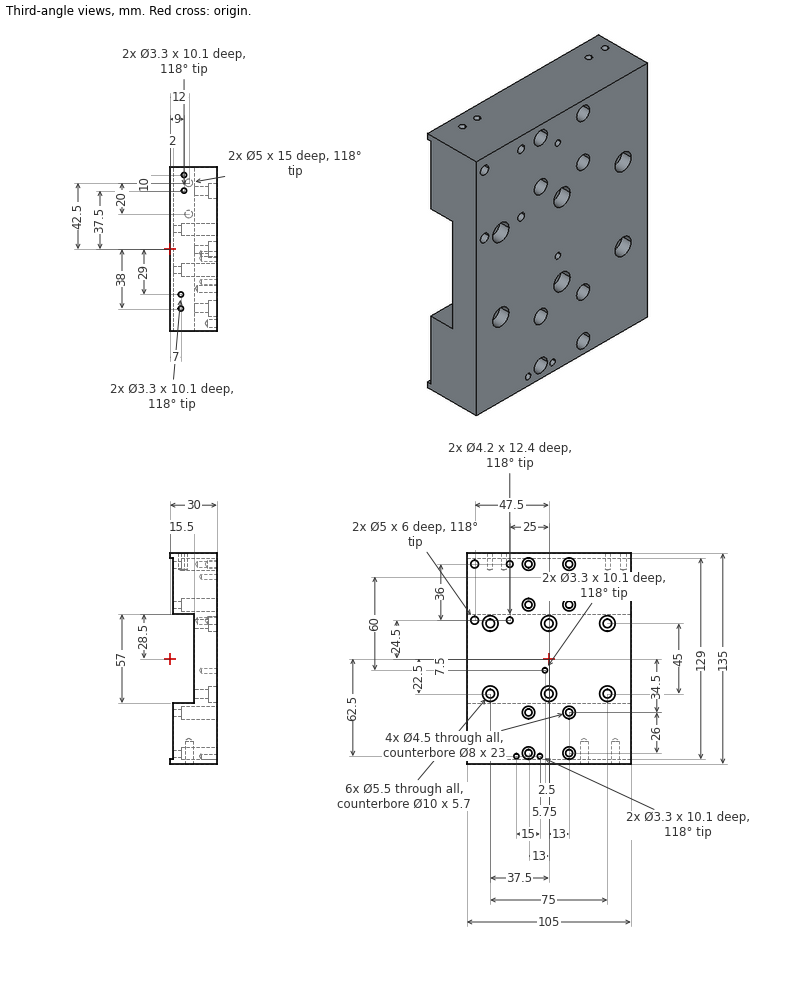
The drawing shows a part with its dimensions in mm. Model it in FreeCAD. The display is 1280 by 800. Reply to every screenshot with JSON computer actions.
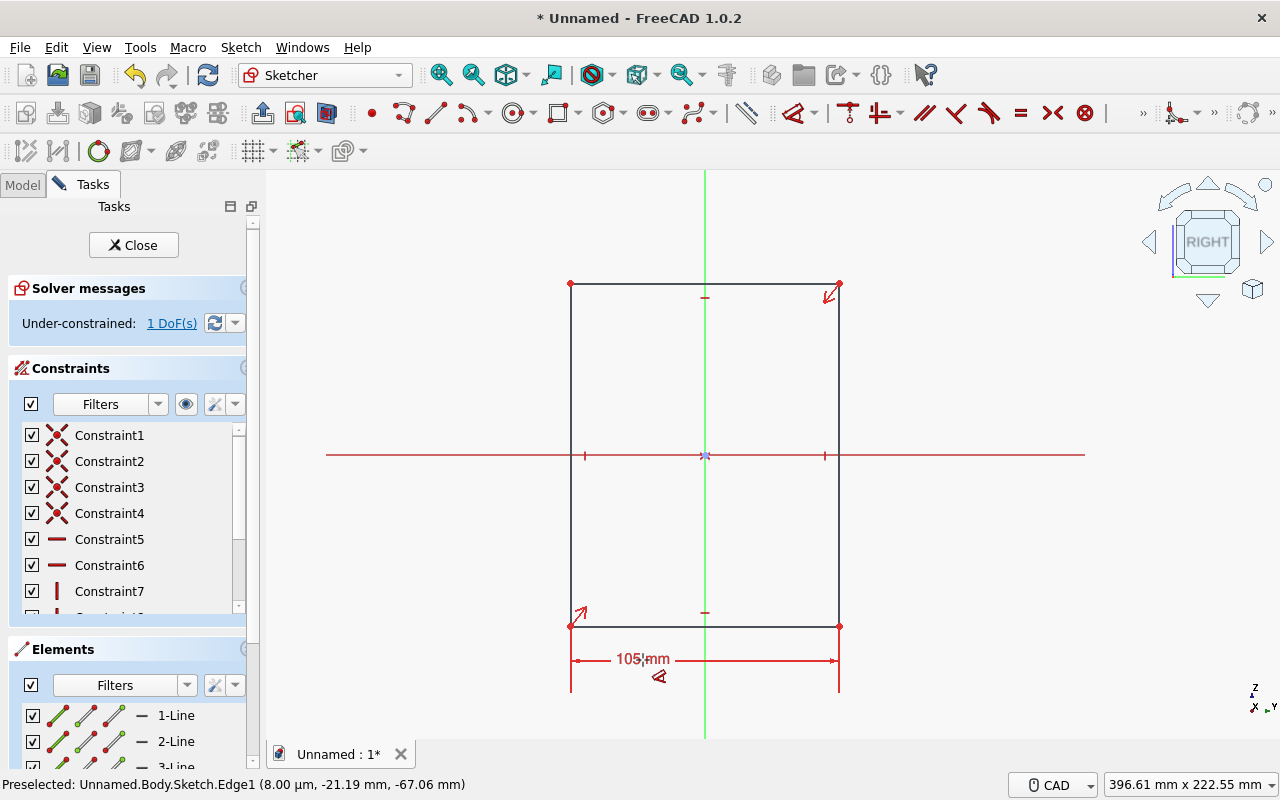
{"action": "left_click", "coordinate": [839, 524]}
{"action": "left_click", "coordinate": [873, 376]}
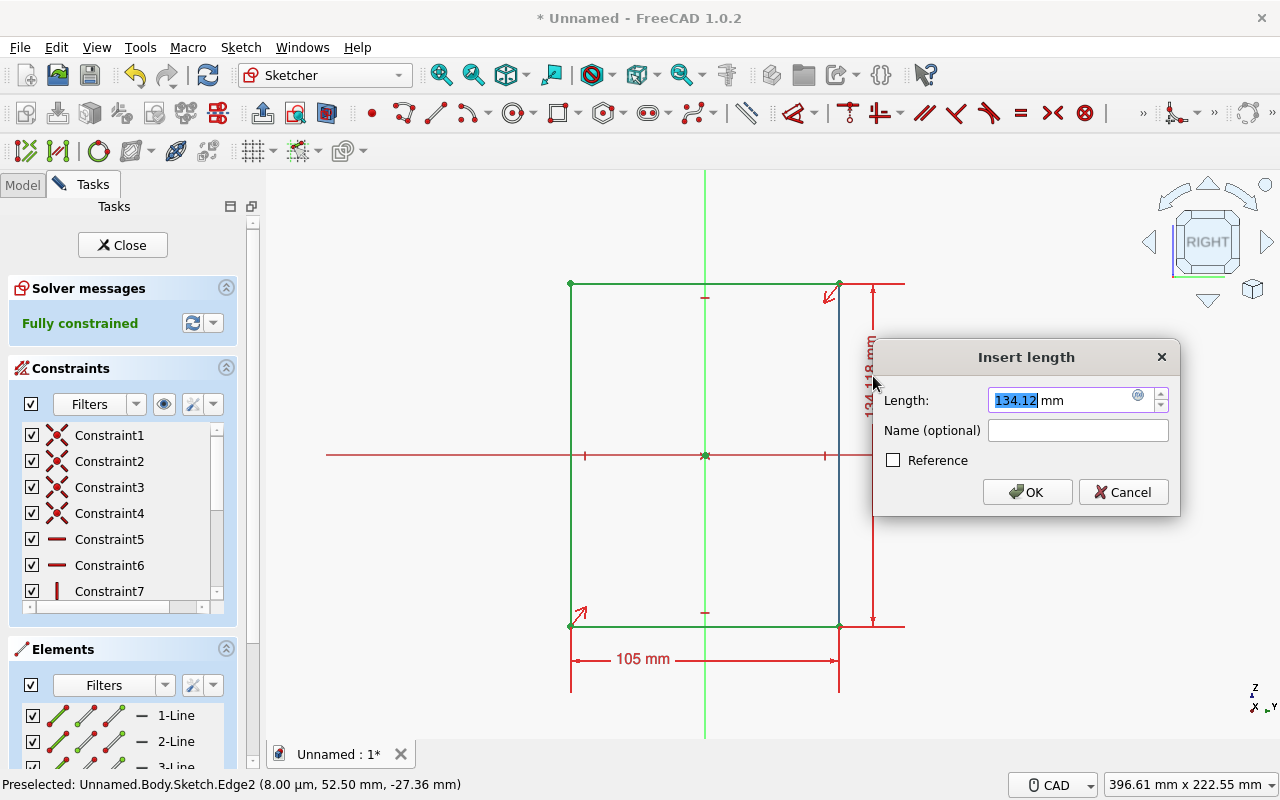
{"action": "type", "text": "135"}
{"action": "key", "text": "Return"}
{"action": "key", "text": "Escape"}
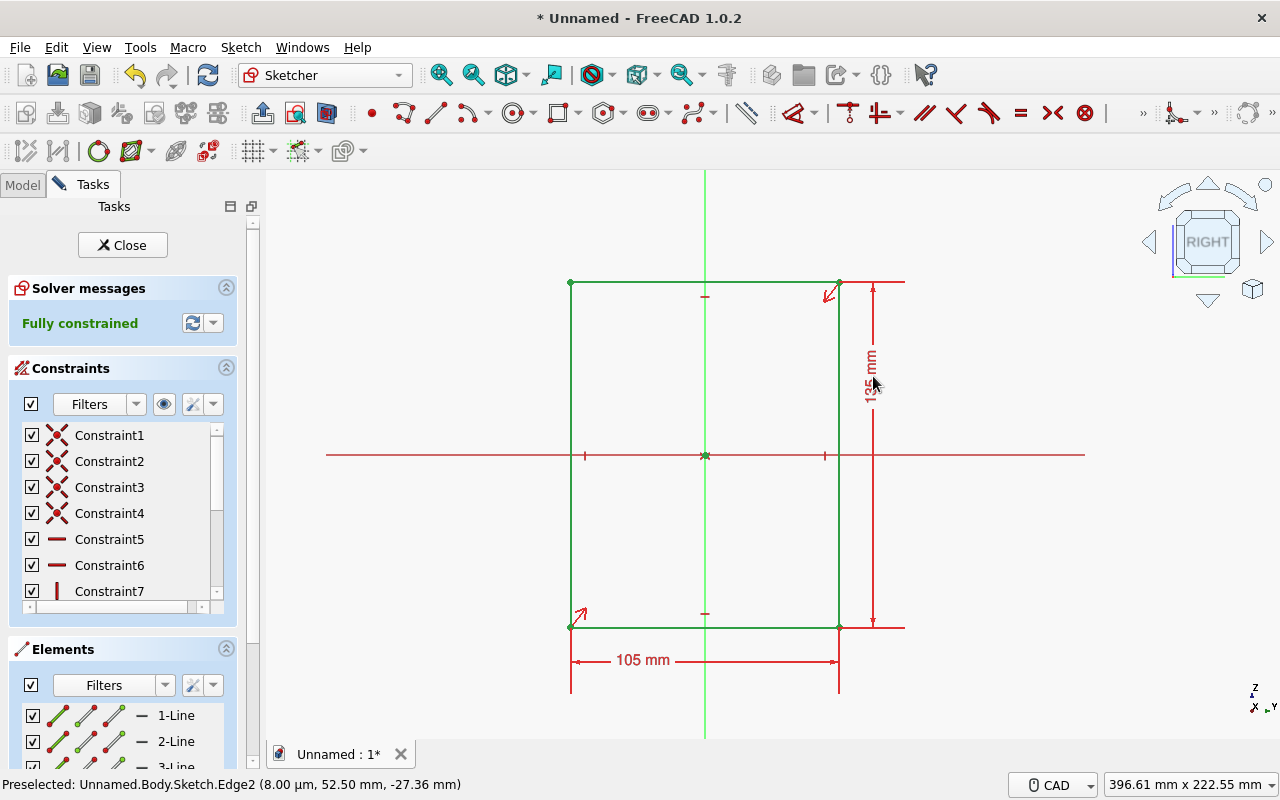
{"action": "left_click", "coordinate": [123, 245]}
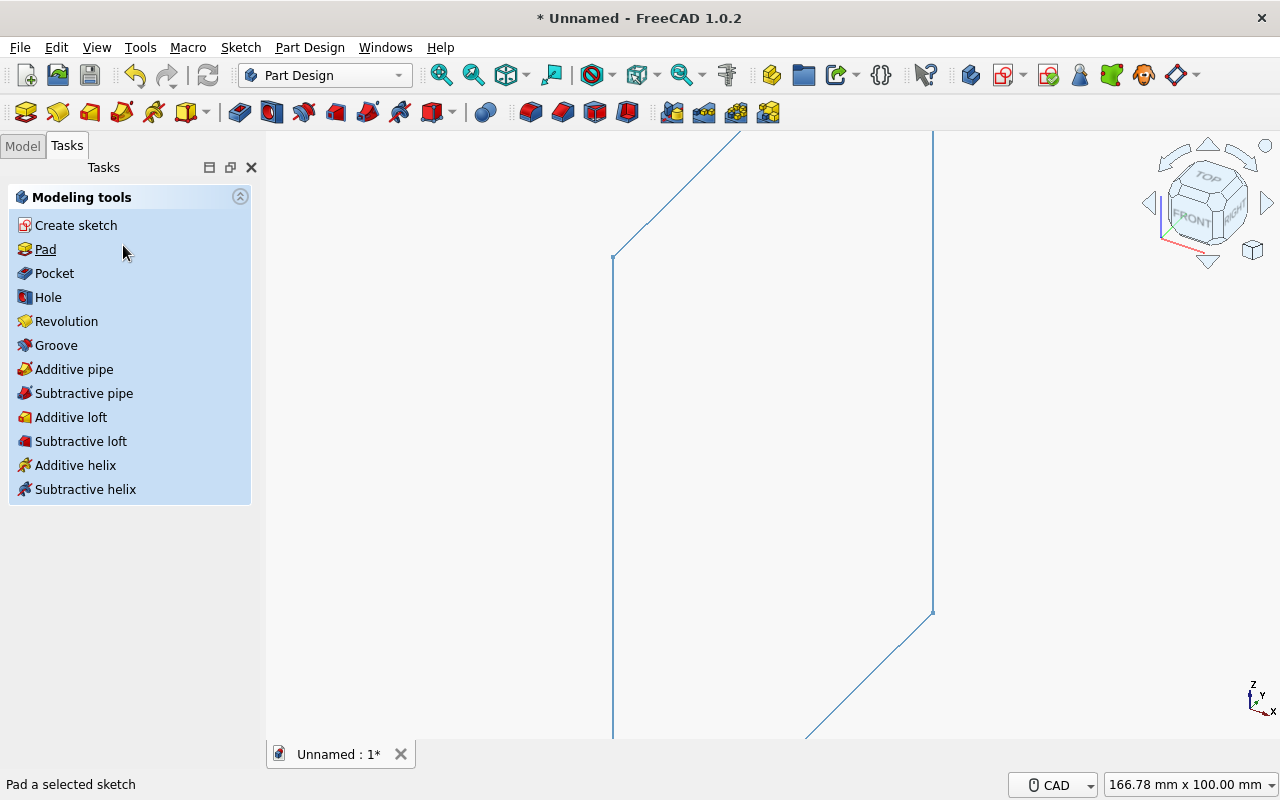
{"action": "left_click", "coordinate": [26, 112]}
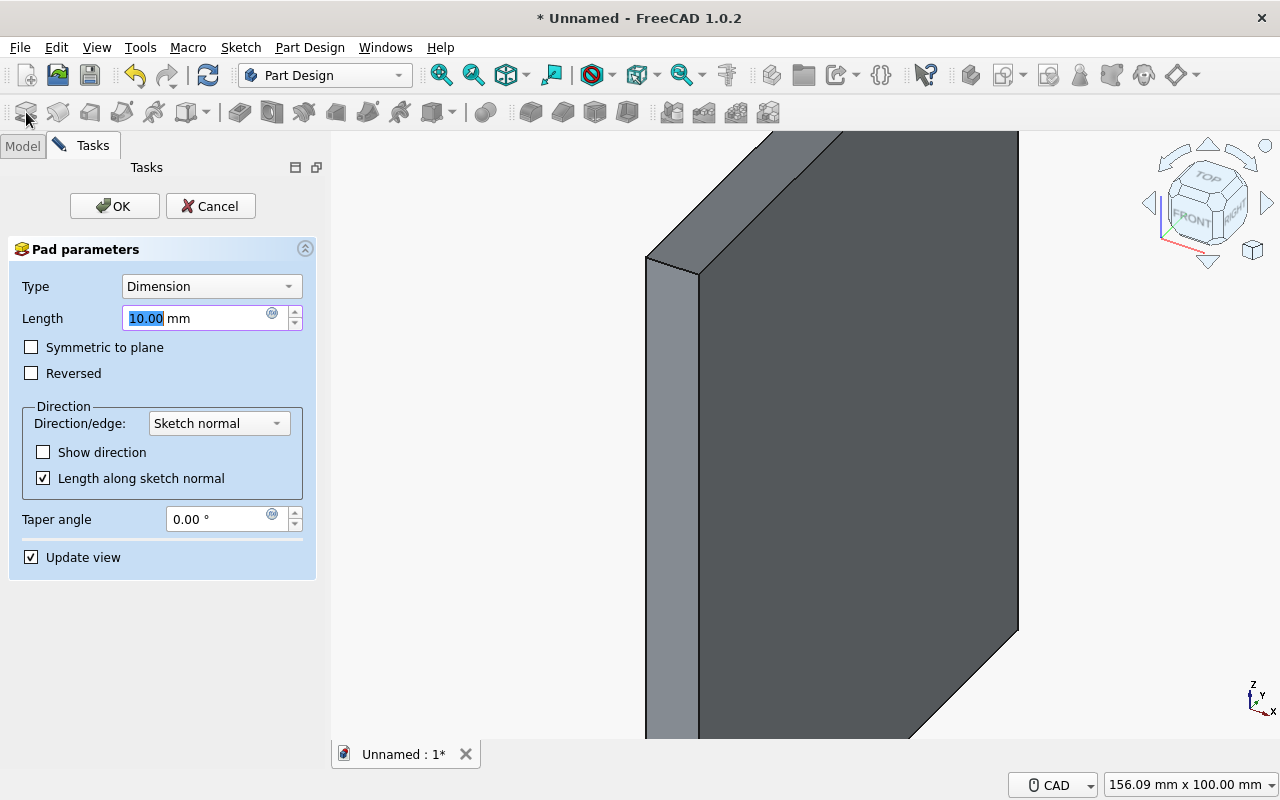
{"action": "type", "text": "30"}
{"action": "key", "text": "Tab"}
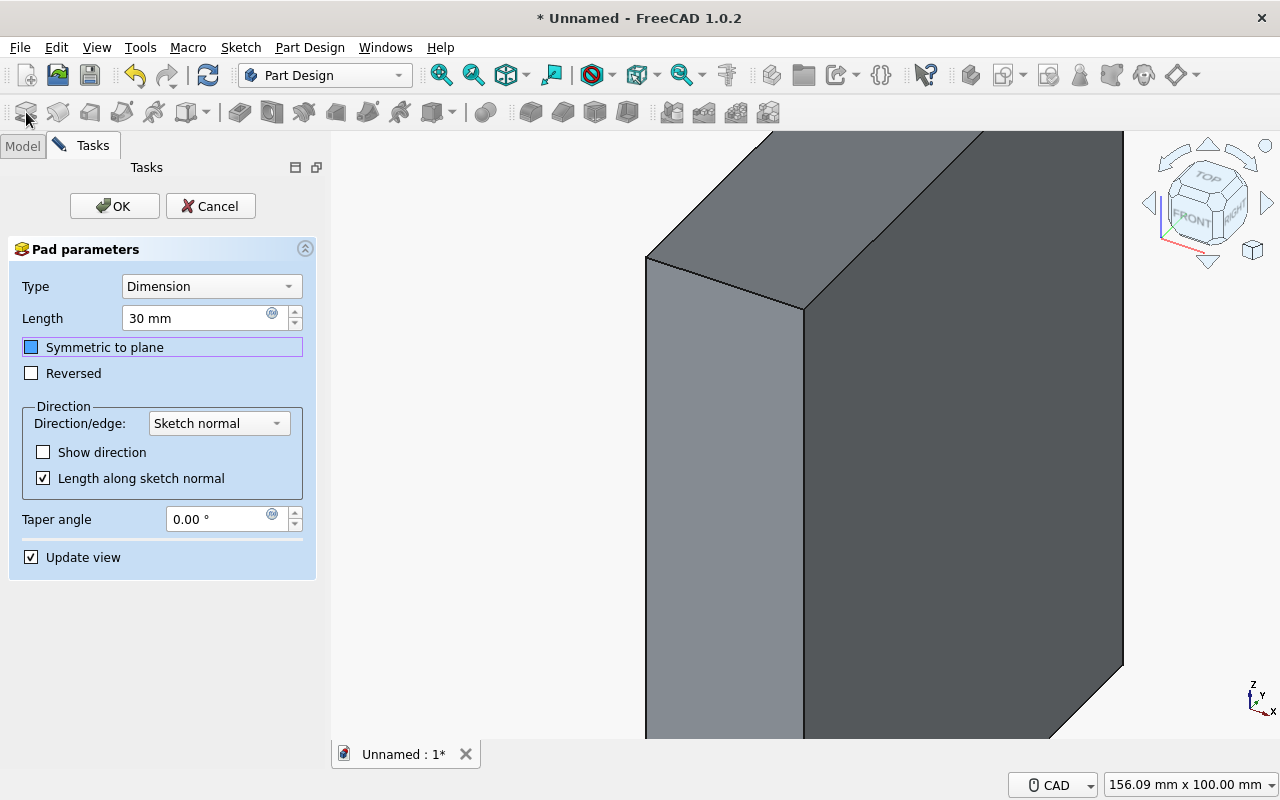
{"action": "left_click", "coordinate": [115, 206]}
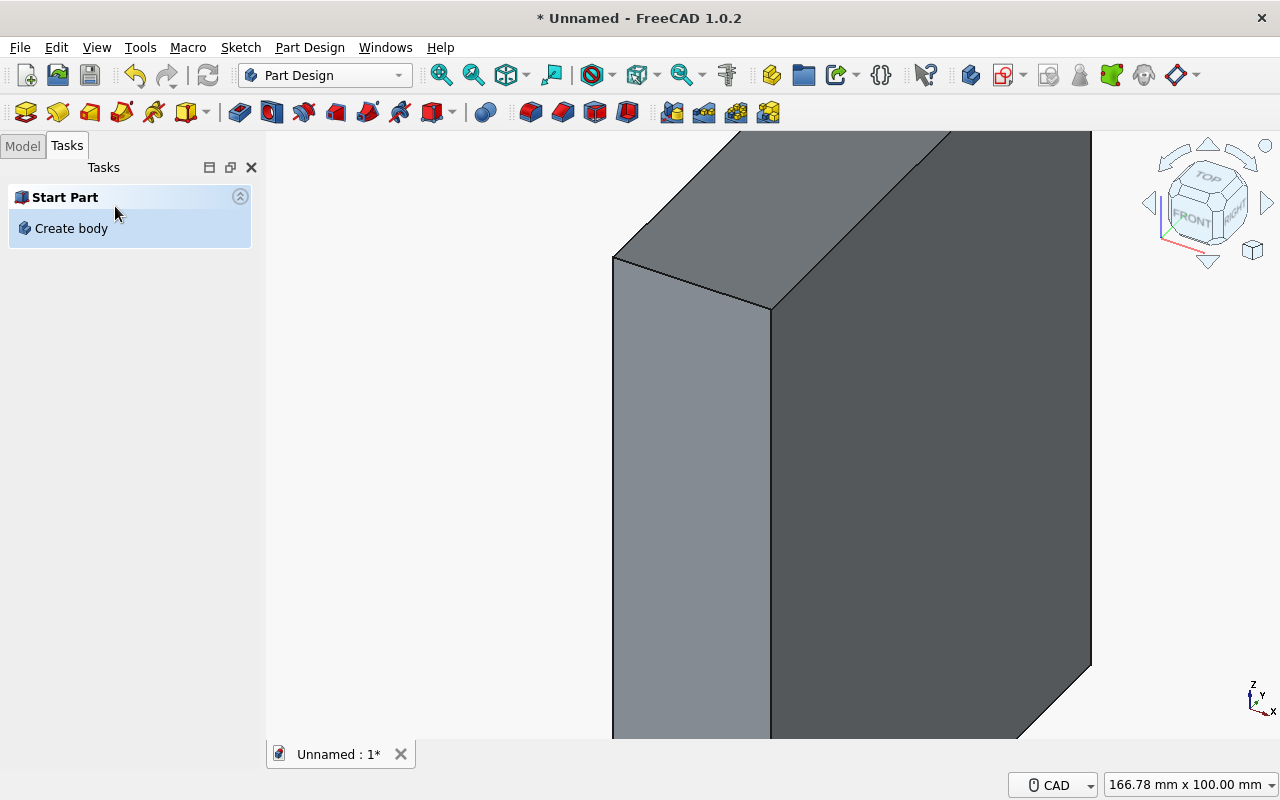
{"action": "left_click", "coordinate": [442, 76]}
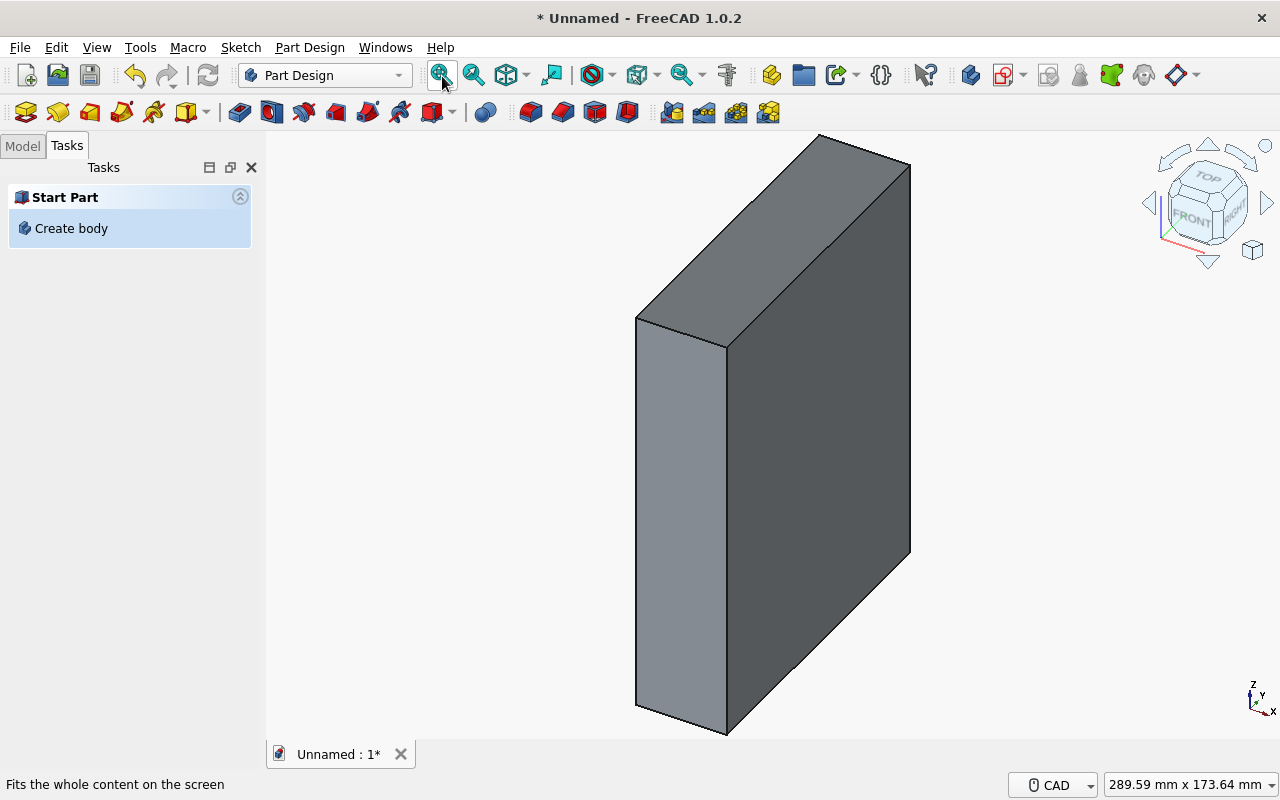
{"action": "left_click", "coordinate": [681, 470]}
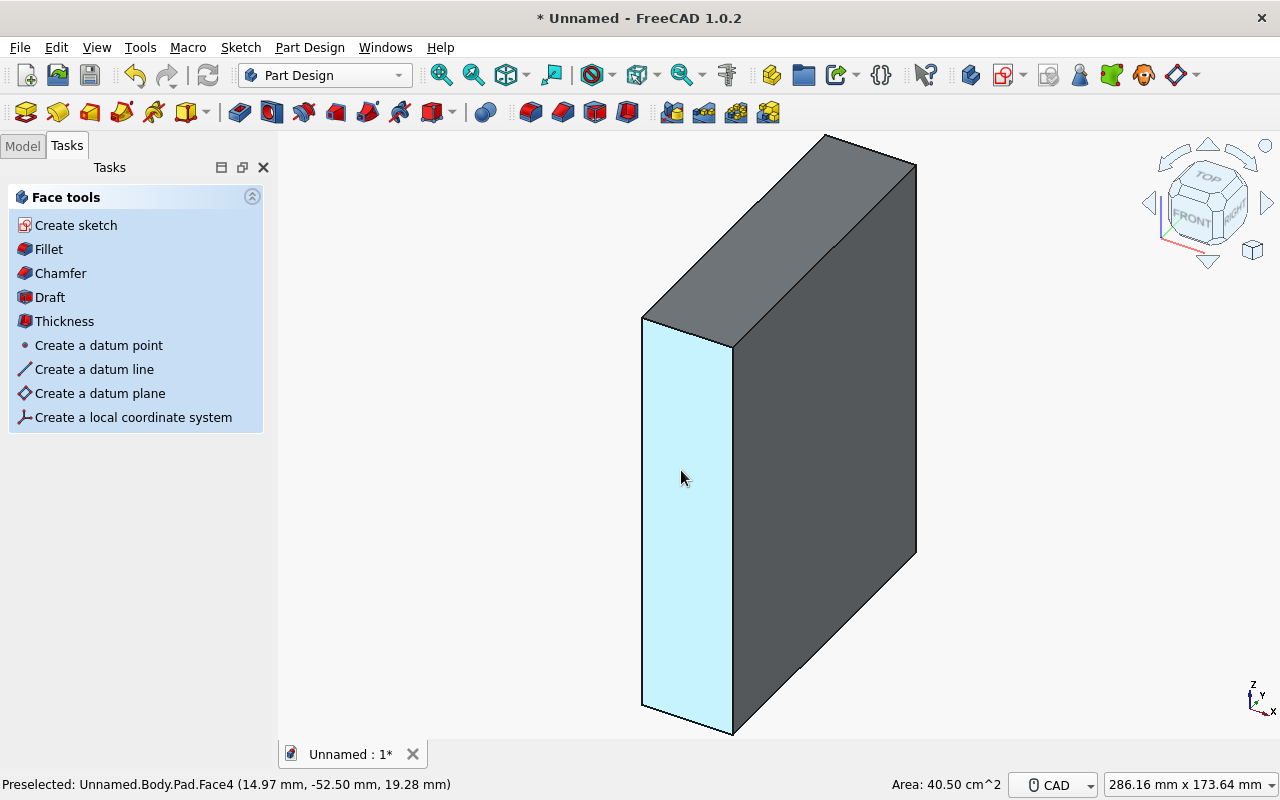
{"action": "left_click", "coordinate": [1004, 76]}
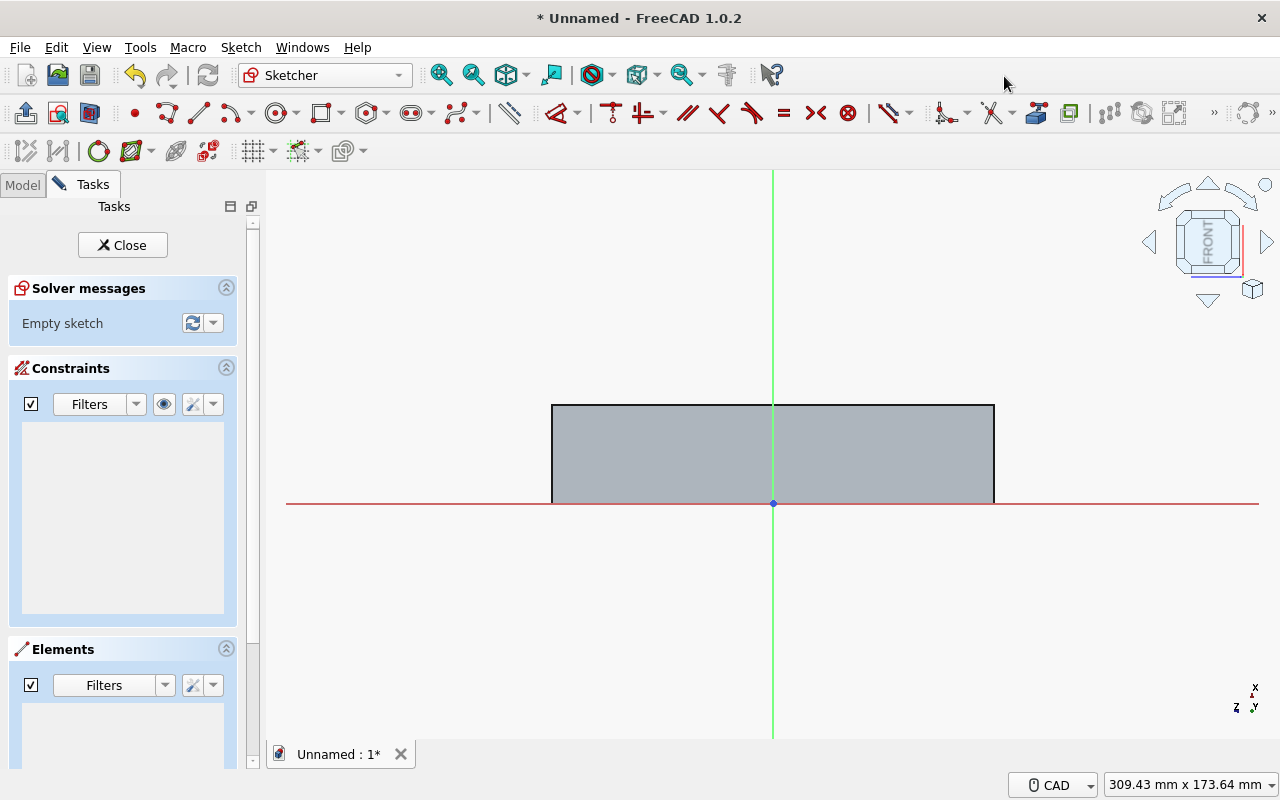
{"action": "scroll", "coordinate": [803, 488], "scroll_direction": "up", "scroll_amount": 6}